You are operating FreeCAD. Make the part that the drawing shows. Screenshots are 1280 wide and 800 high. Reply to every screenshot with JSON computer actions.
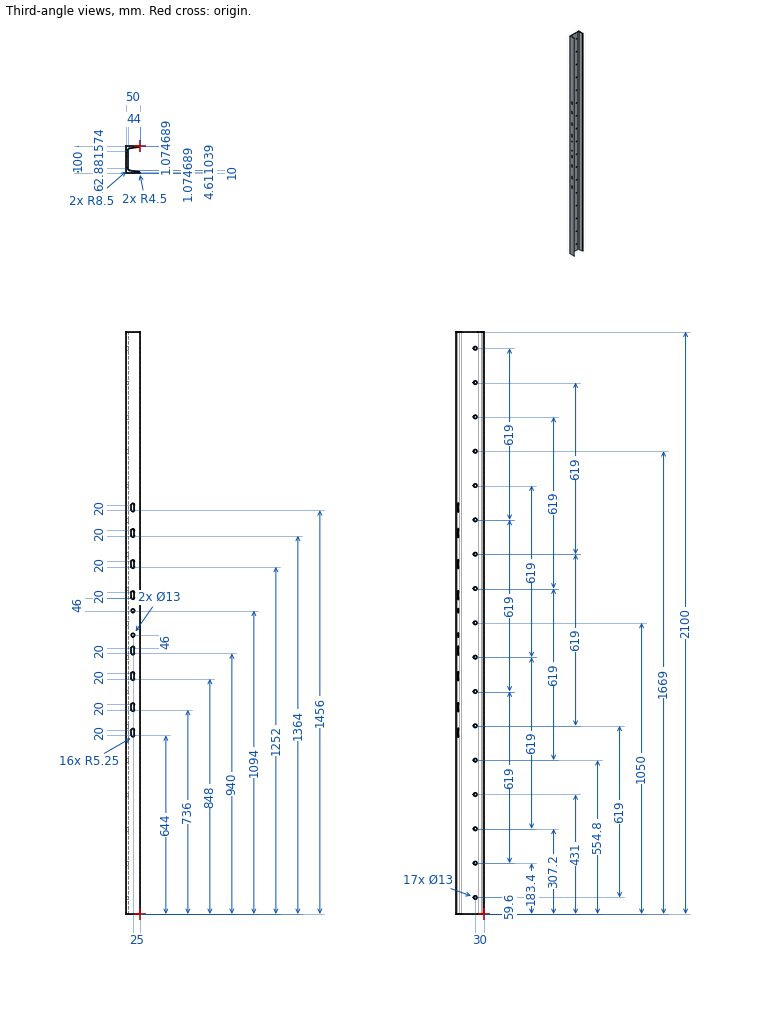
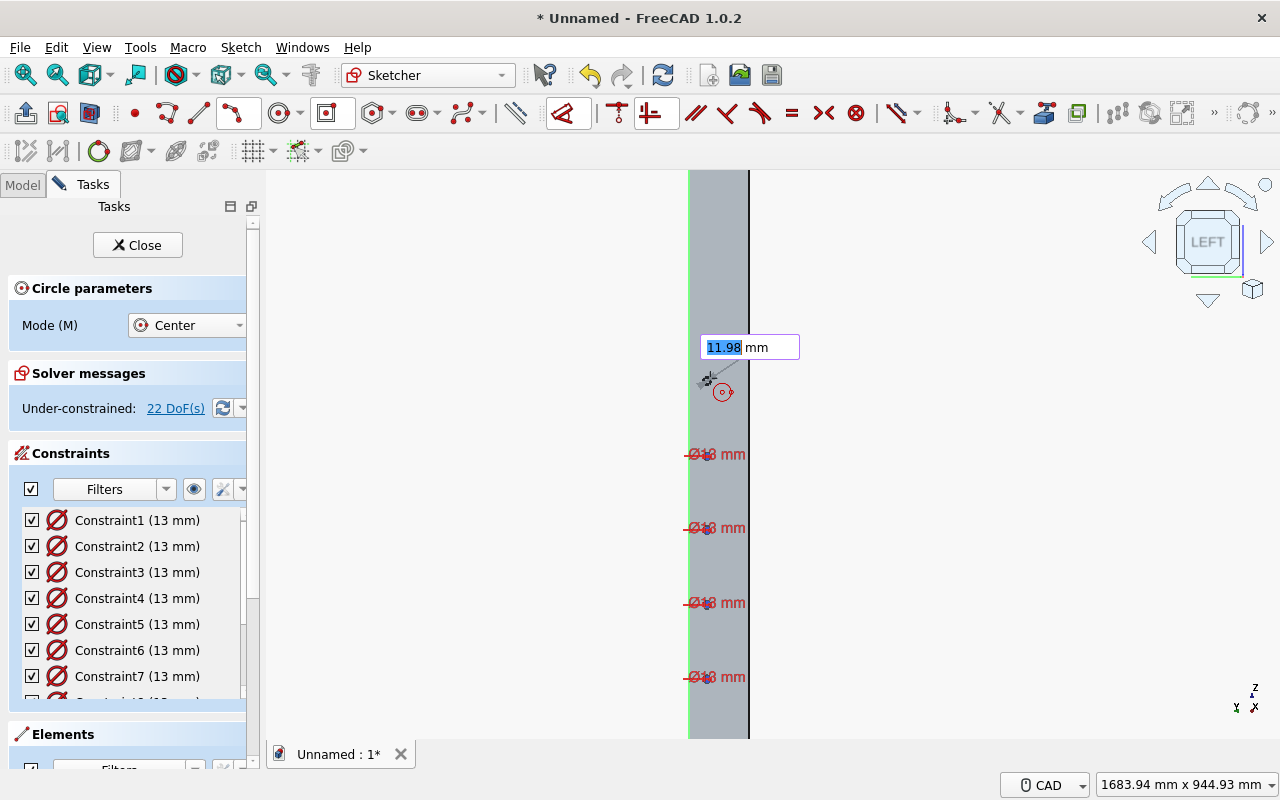
{"action": "type", "text": "13"}
{"action": "key", "text": "Return"}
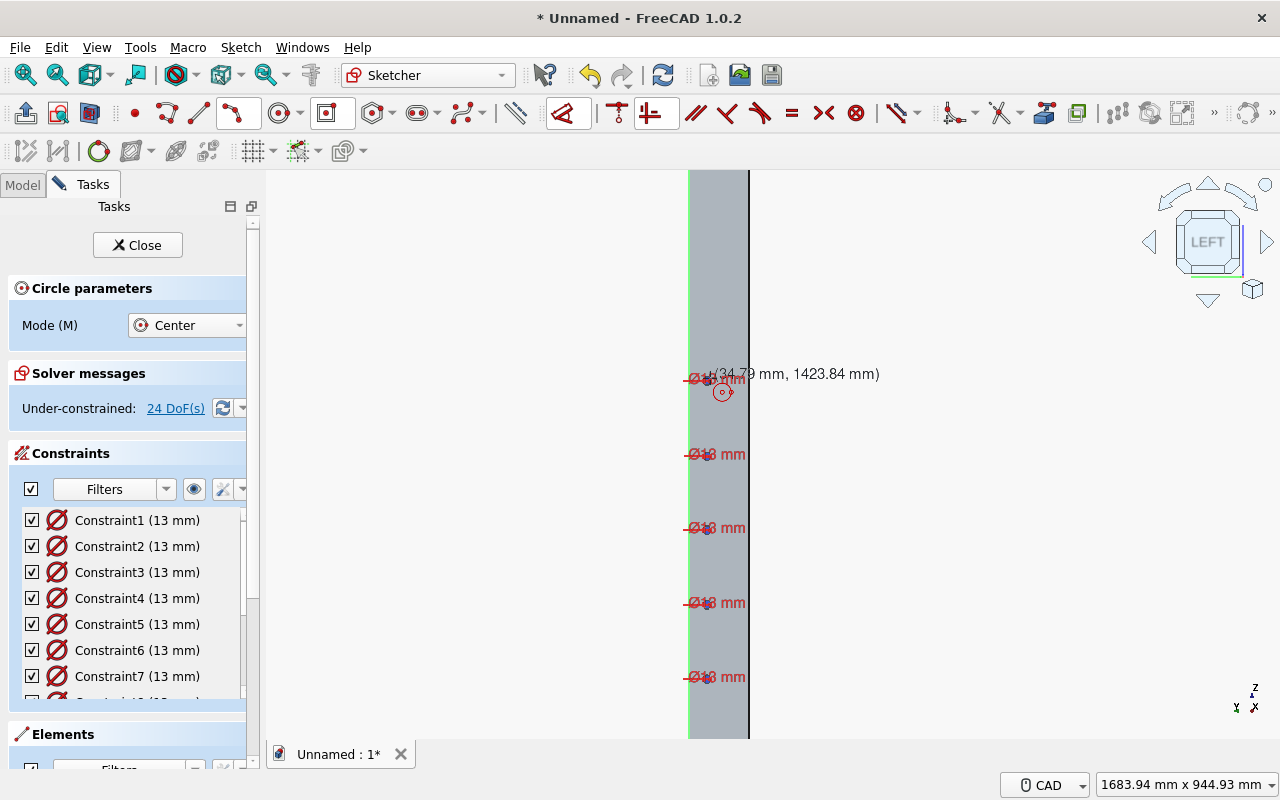
{"action": "scroll", "coordinate": [707, 306], "scroll_direction": "up", "scroll_amount": 9}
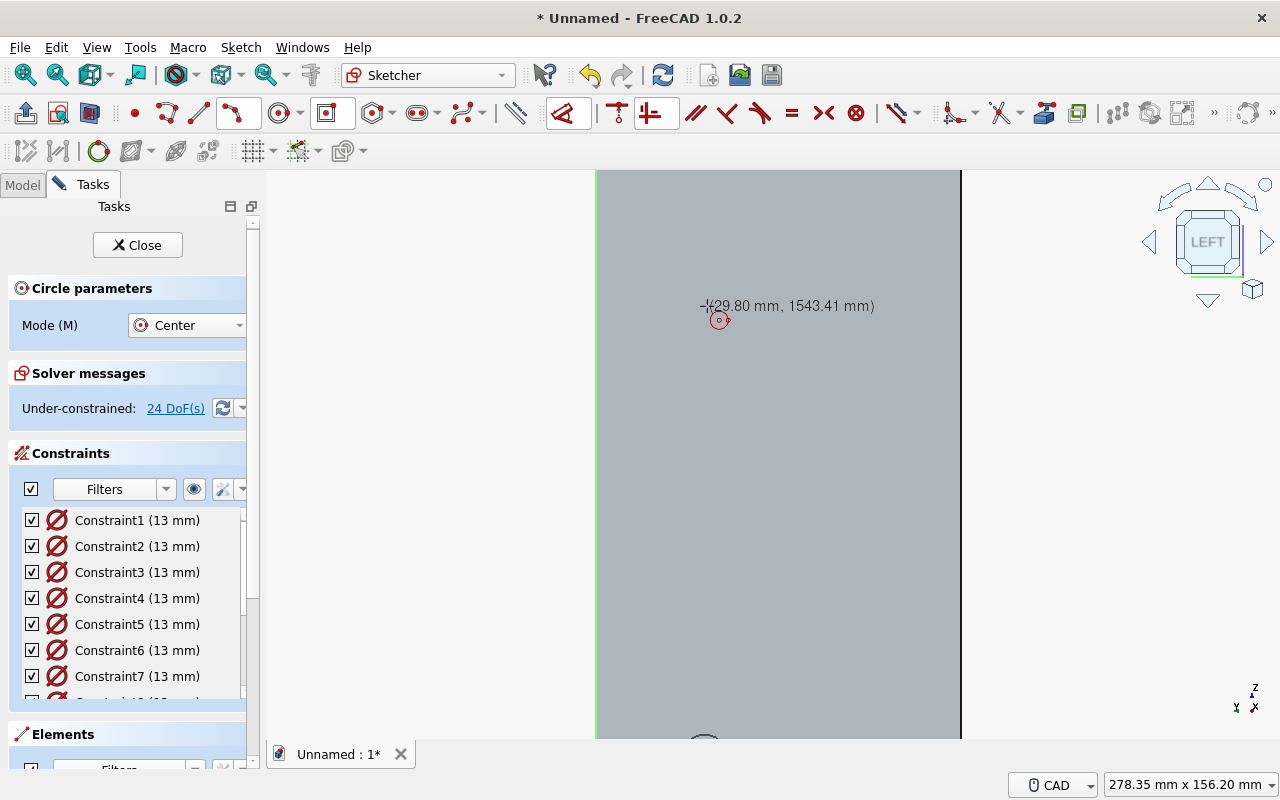
{"action": "scroll", "coordinate": [707, 363], "scroll_direction": "down", "scroll_amount": 15}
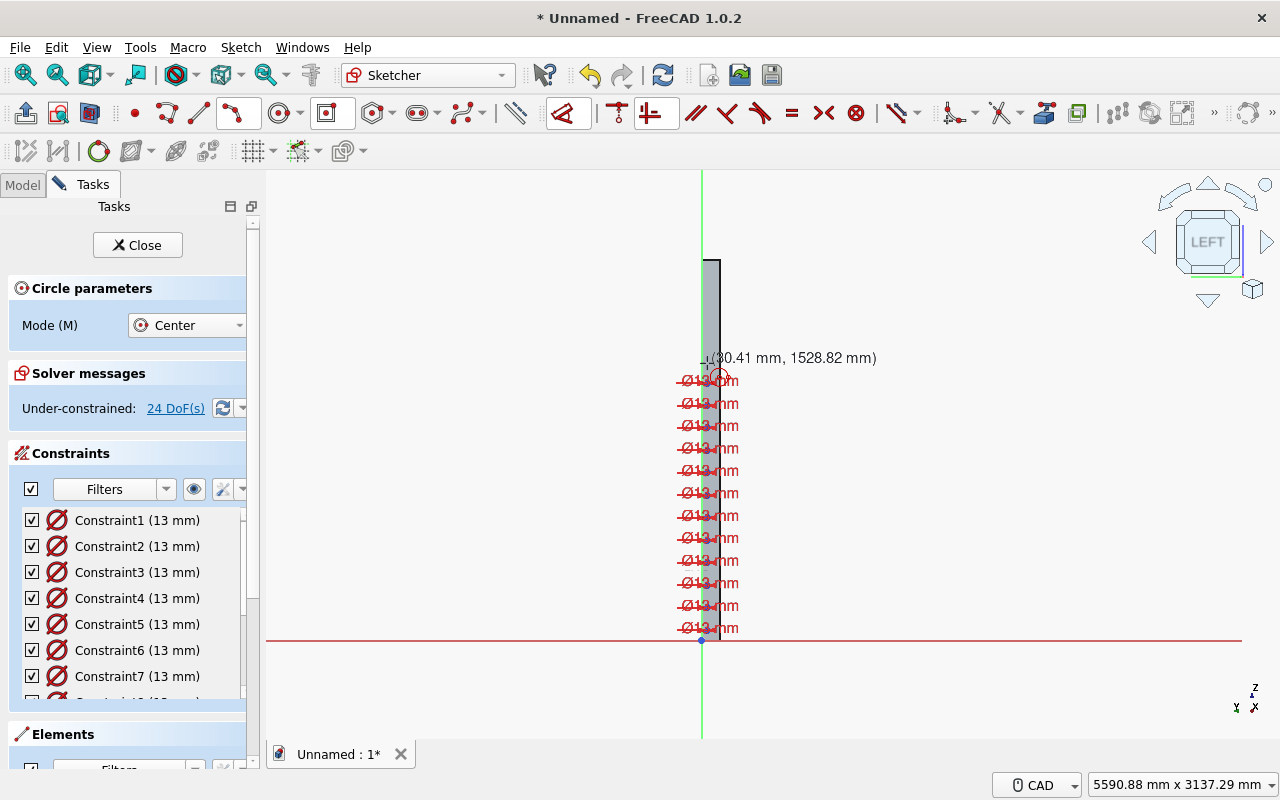
{"action": "scroll", "coordinate": [707, 360], "scroll_direction": "up", "scroll_amount": 6}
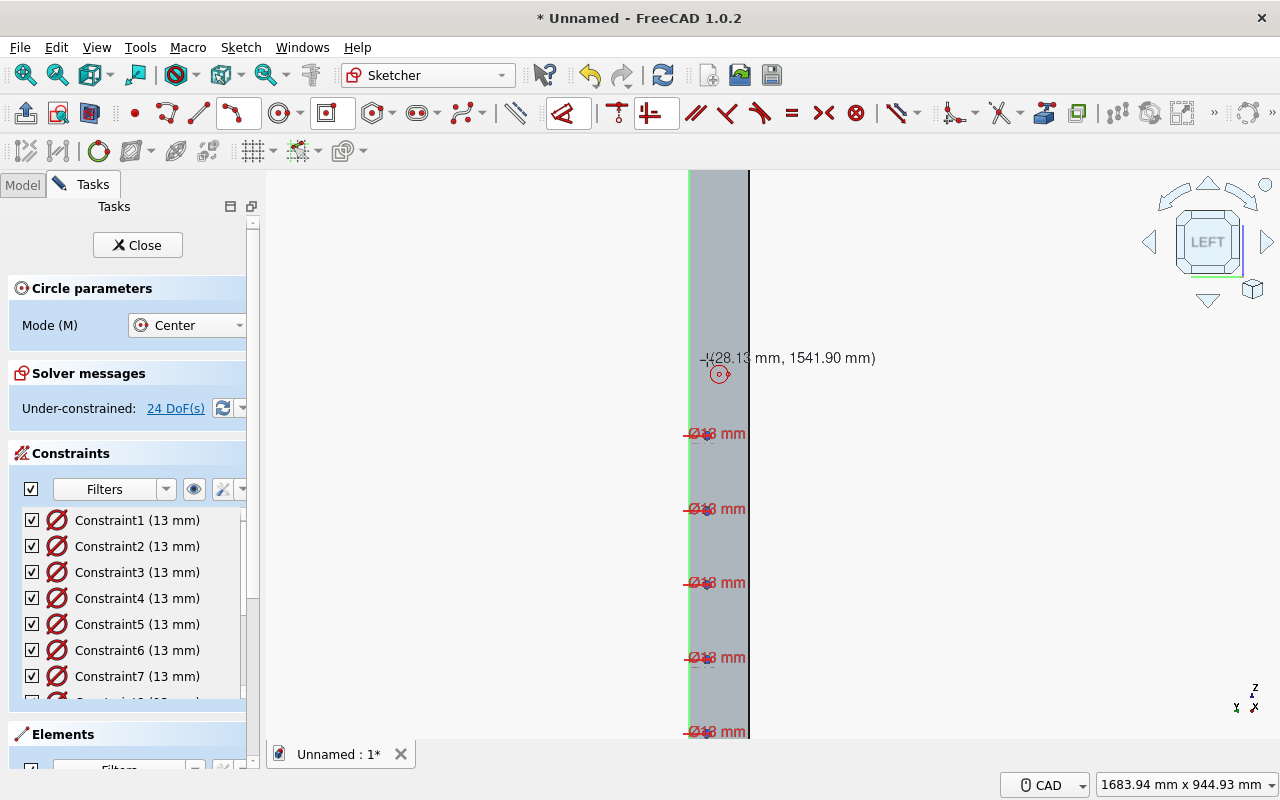
{"action": "left_click", "coordinate": [707, 361]}
{"action": "mouse_move", "coordinate": [710, 358]}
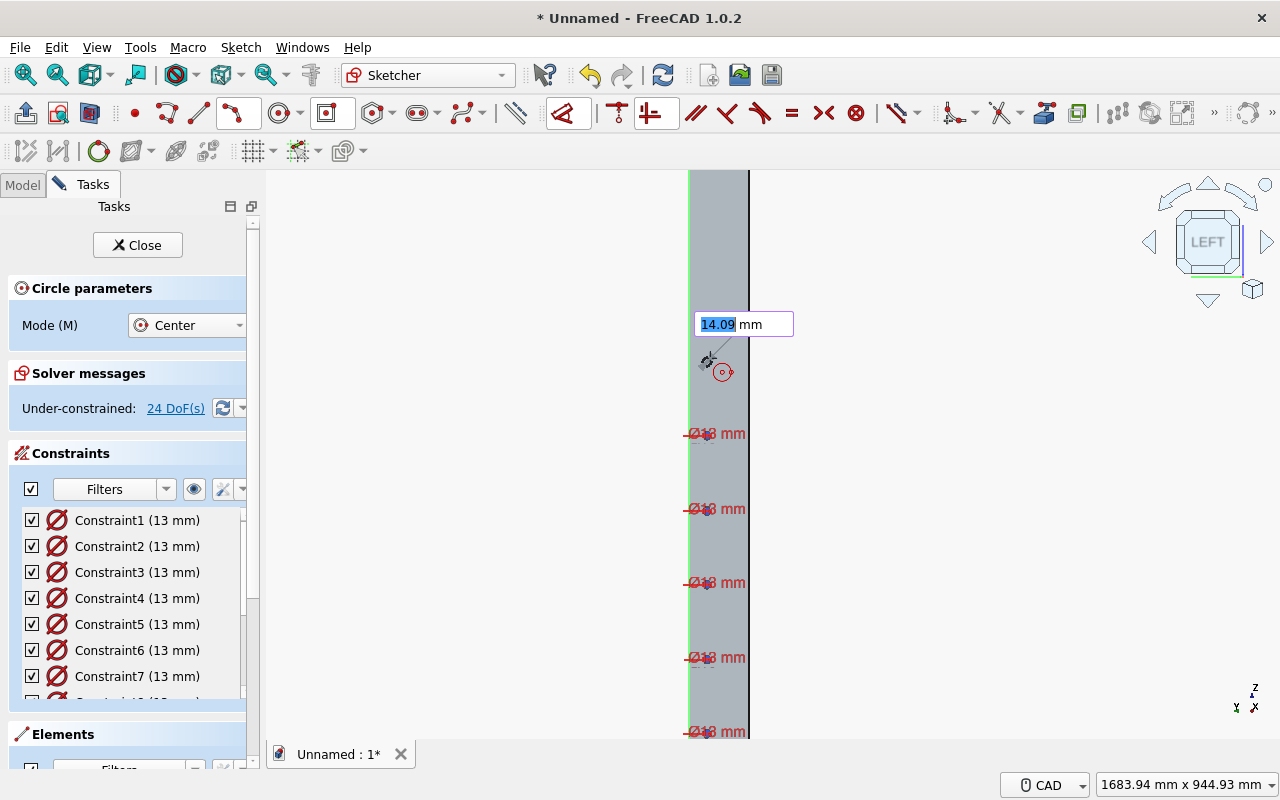
{"action": "type", "text": "13"}
{"action": "key", "text": "Return"}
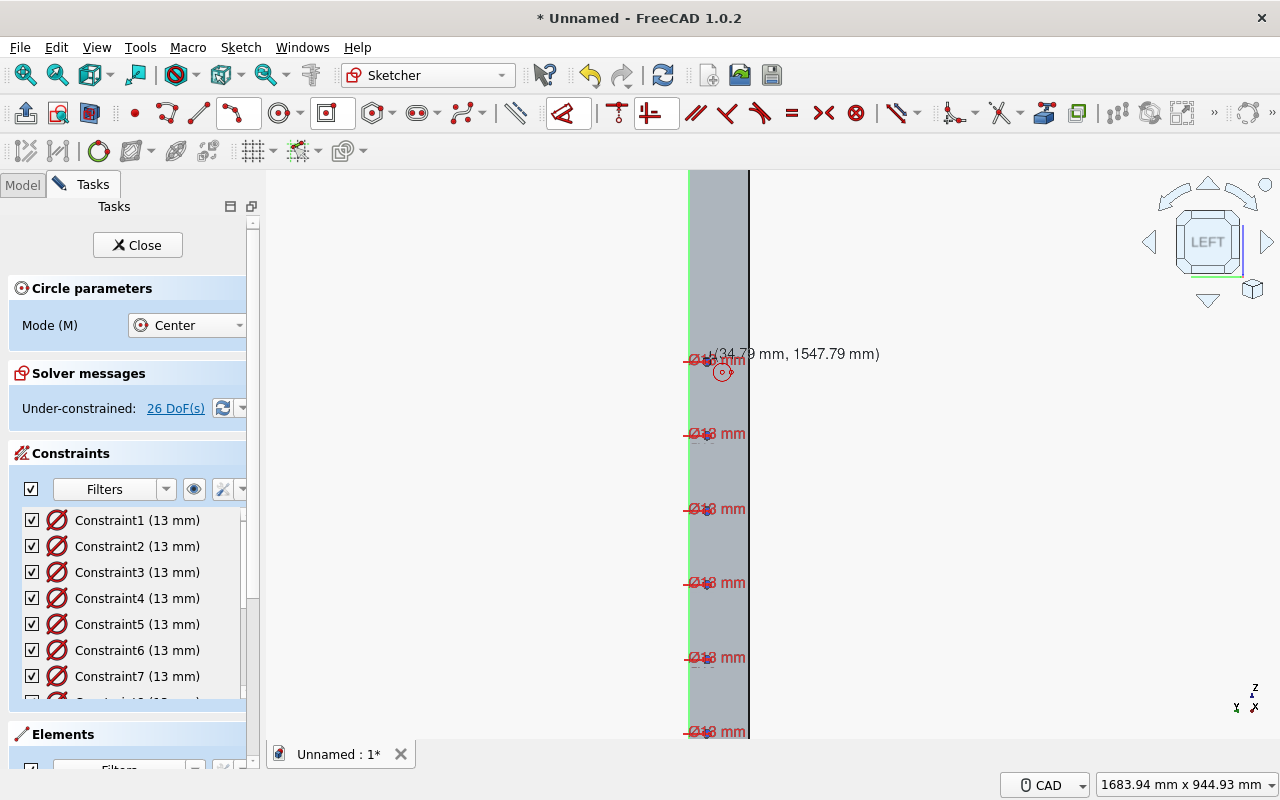
{"action": "scroll", "coordinate": [707, 286], "scroll_direction": "up", "scroll_amount": 9}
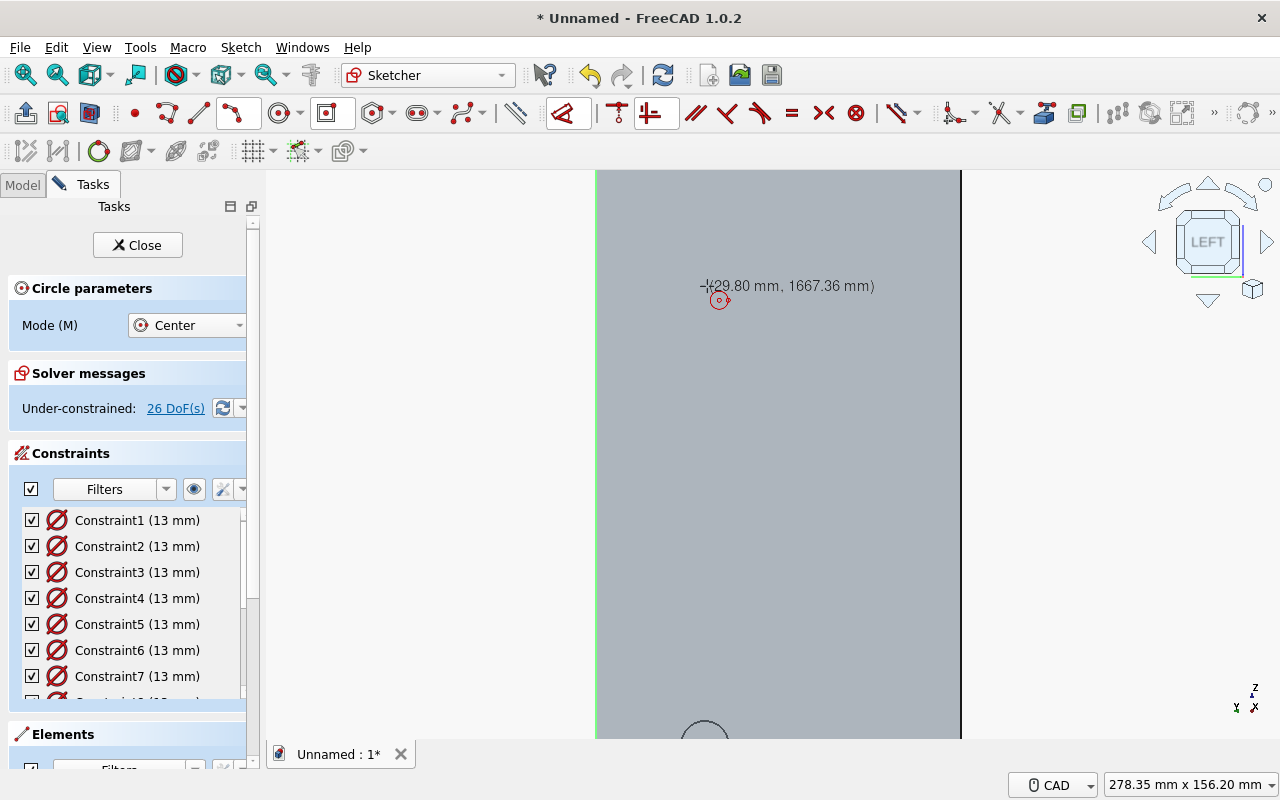
{"action": "scroll", "coordinate": [707, 340], "scroll_direction": "down", "scroll_amount": 15}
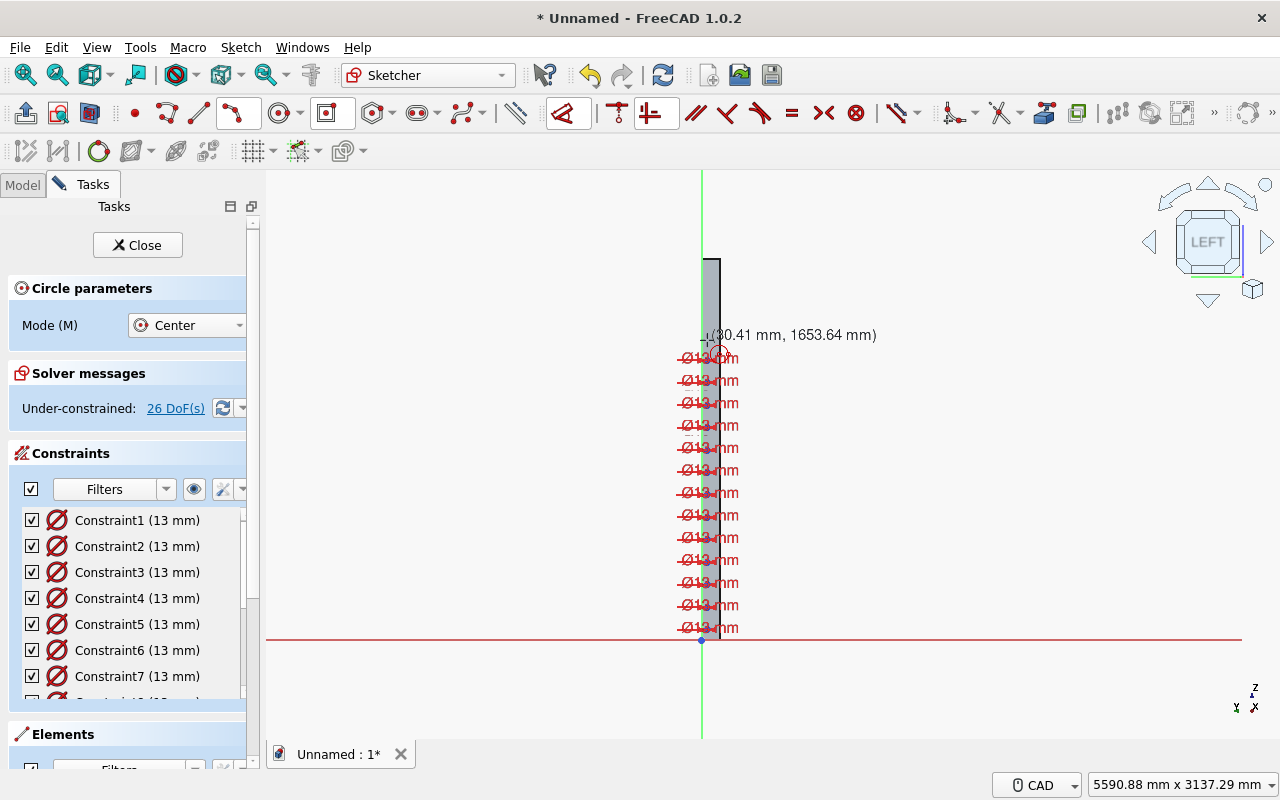
{"action": "scroll", "coordinate": [707, 338], "scroll_direction": "up", "scroll_amount": 6}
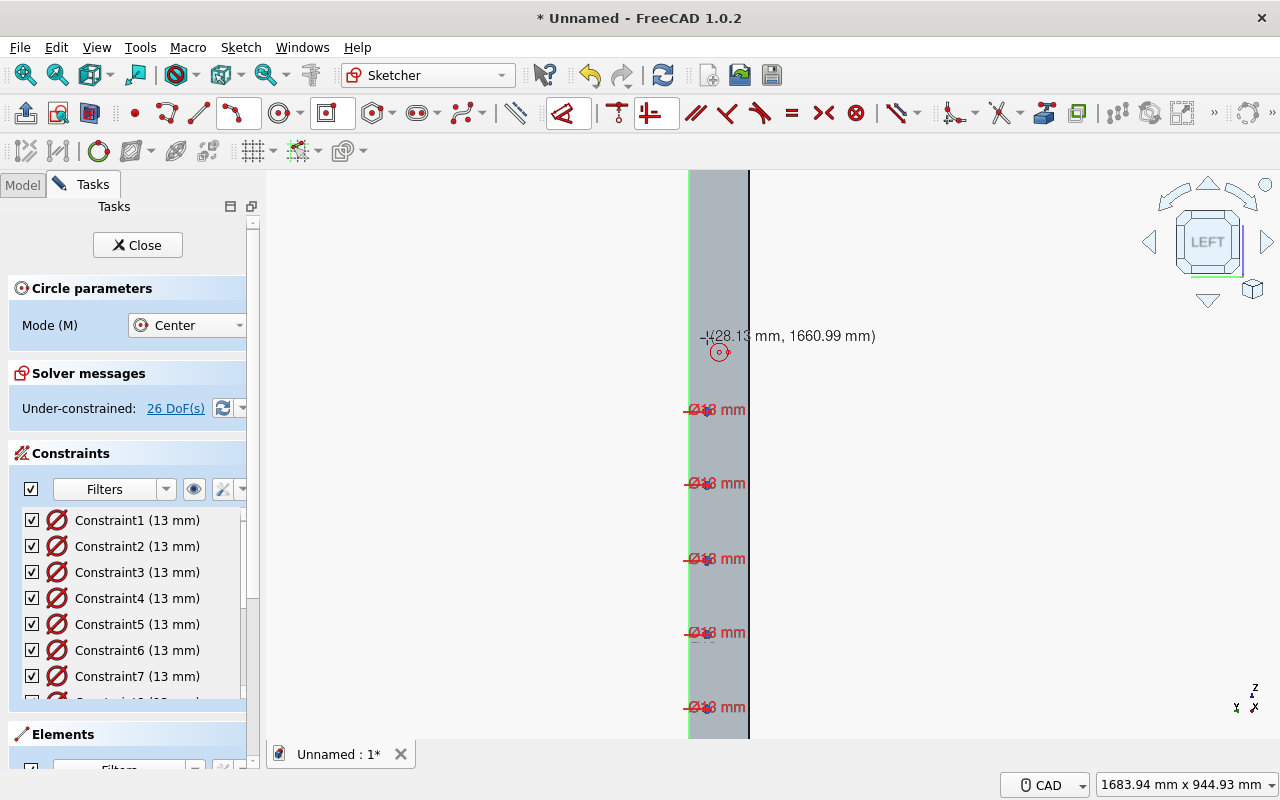
{"action": "left_click", "coordinate": [707, 336]}
{"action": "mouse_move", "coordinate": [710, 333]}